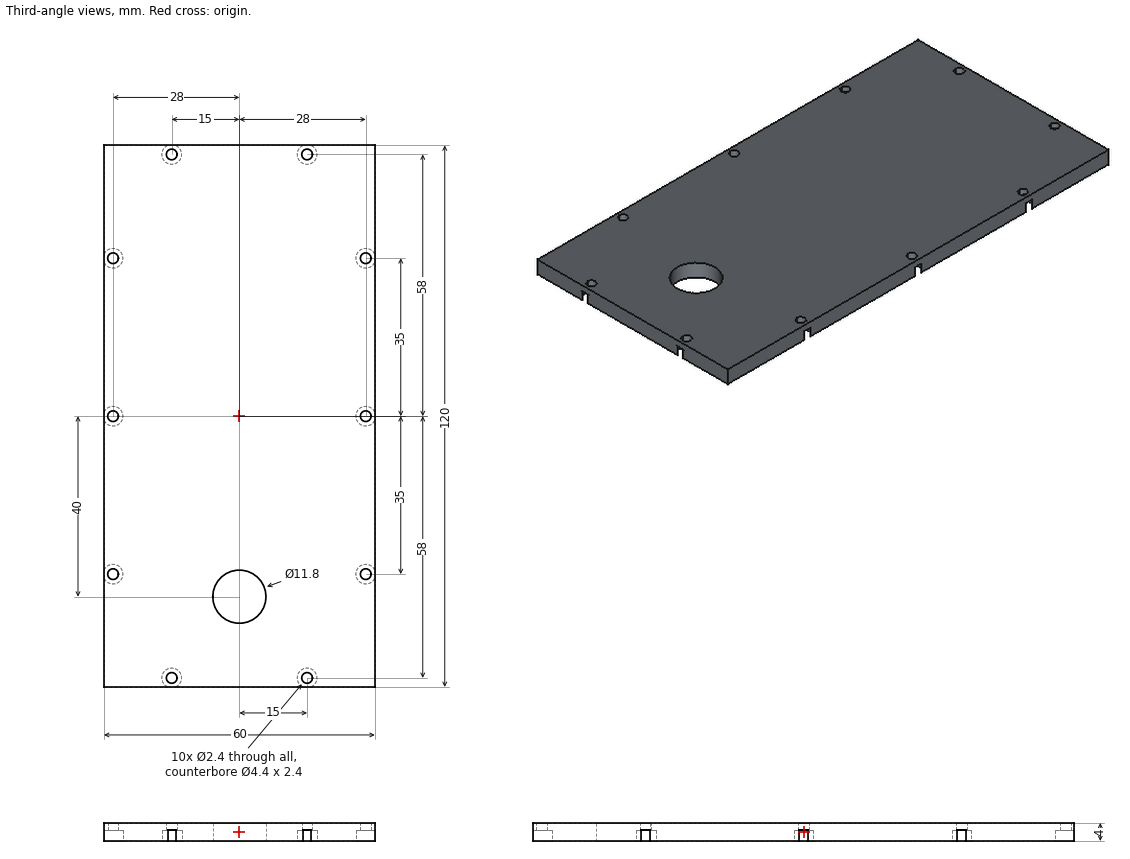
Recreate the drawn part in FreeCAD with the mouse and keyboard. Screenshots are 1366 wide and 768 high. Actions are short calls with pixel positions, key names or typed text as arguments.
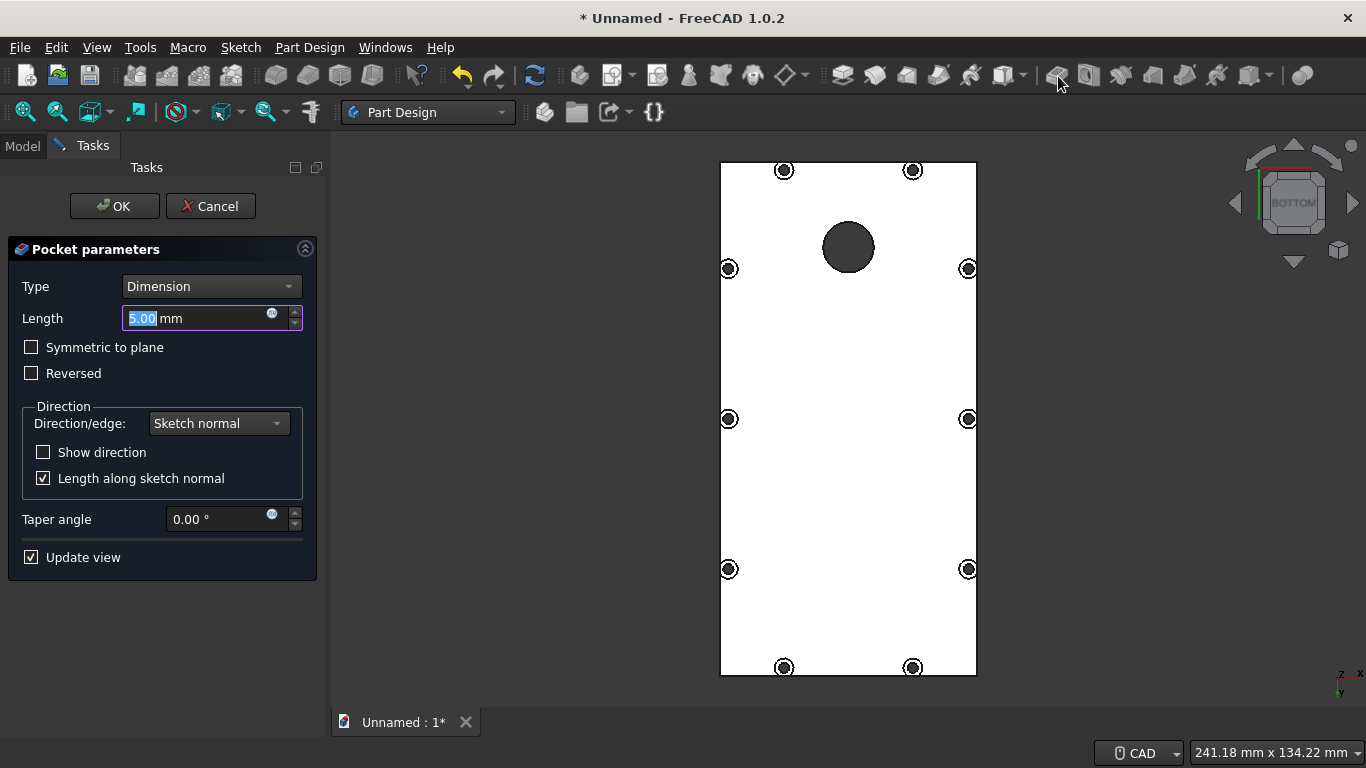
click(212, 286)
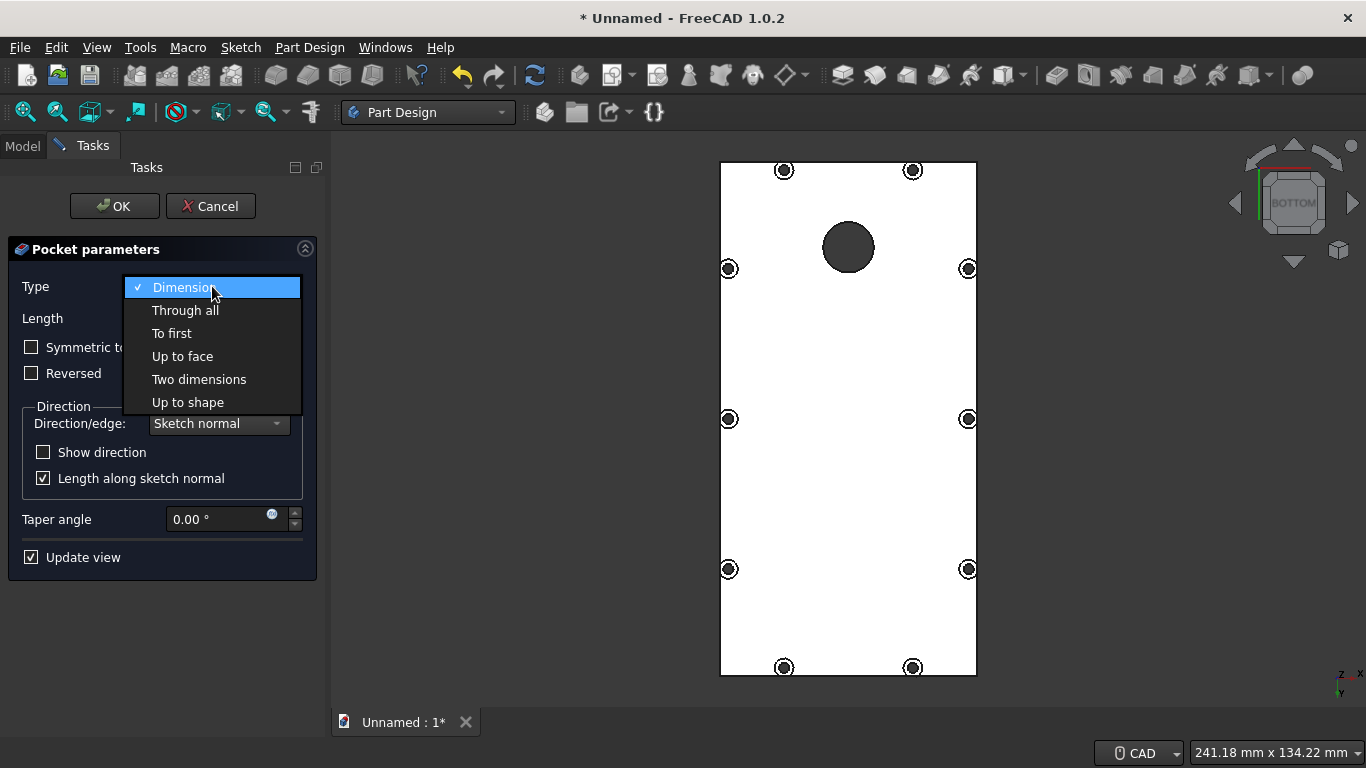
click(212, 310)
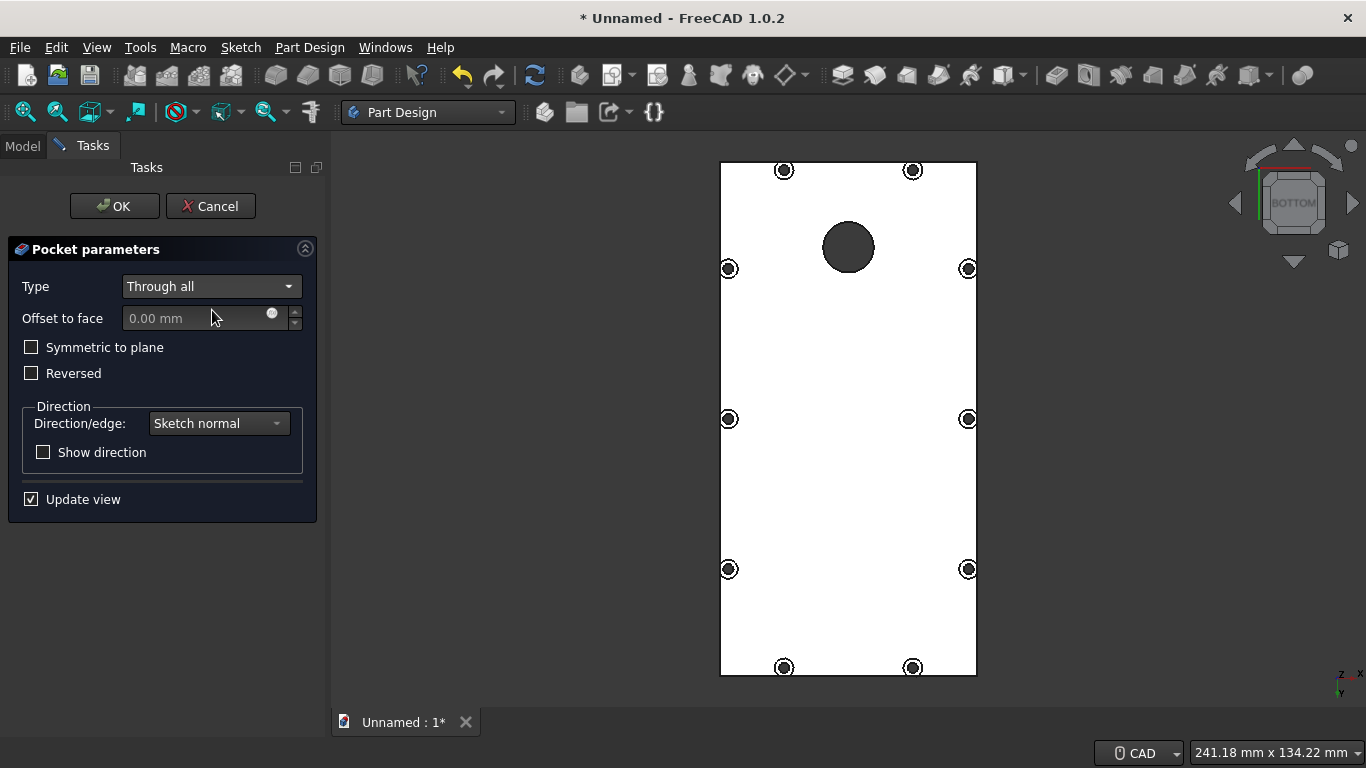
click(115, 206)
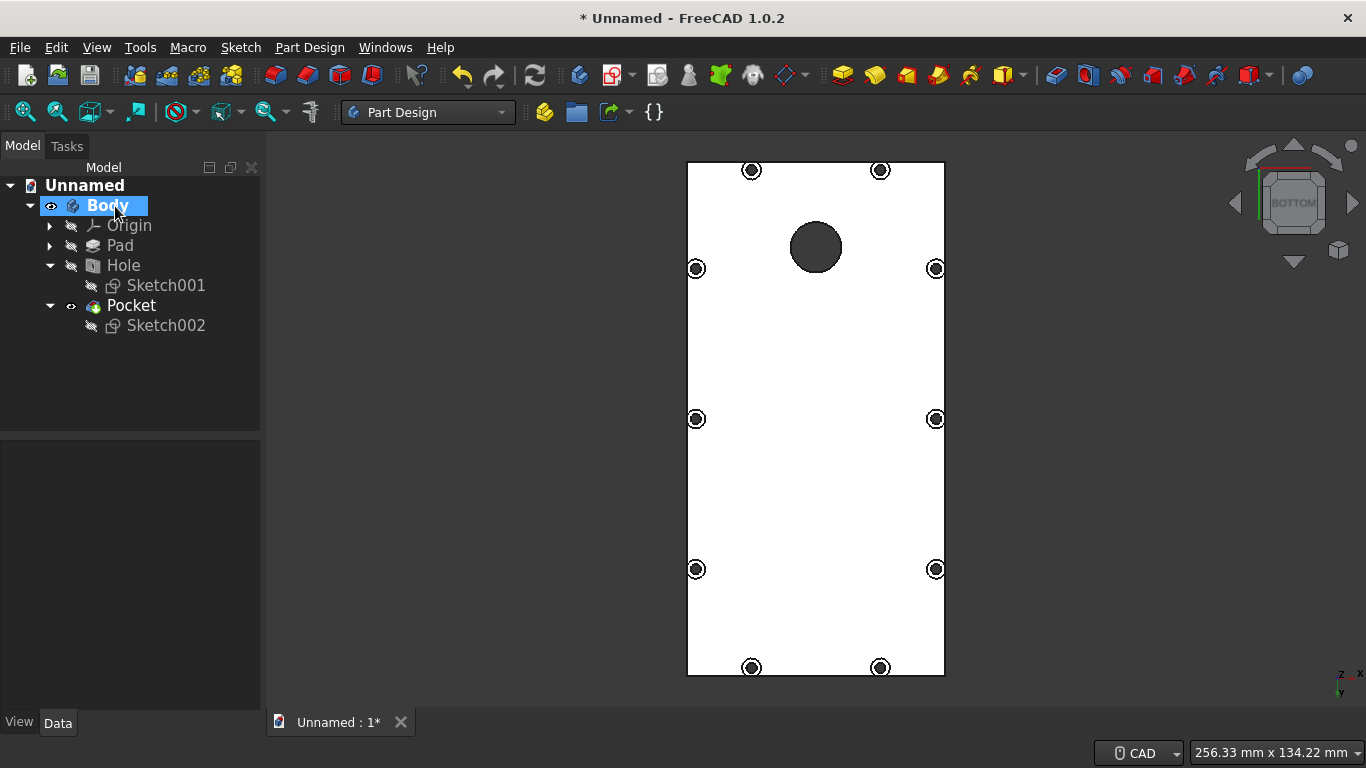
key(0)